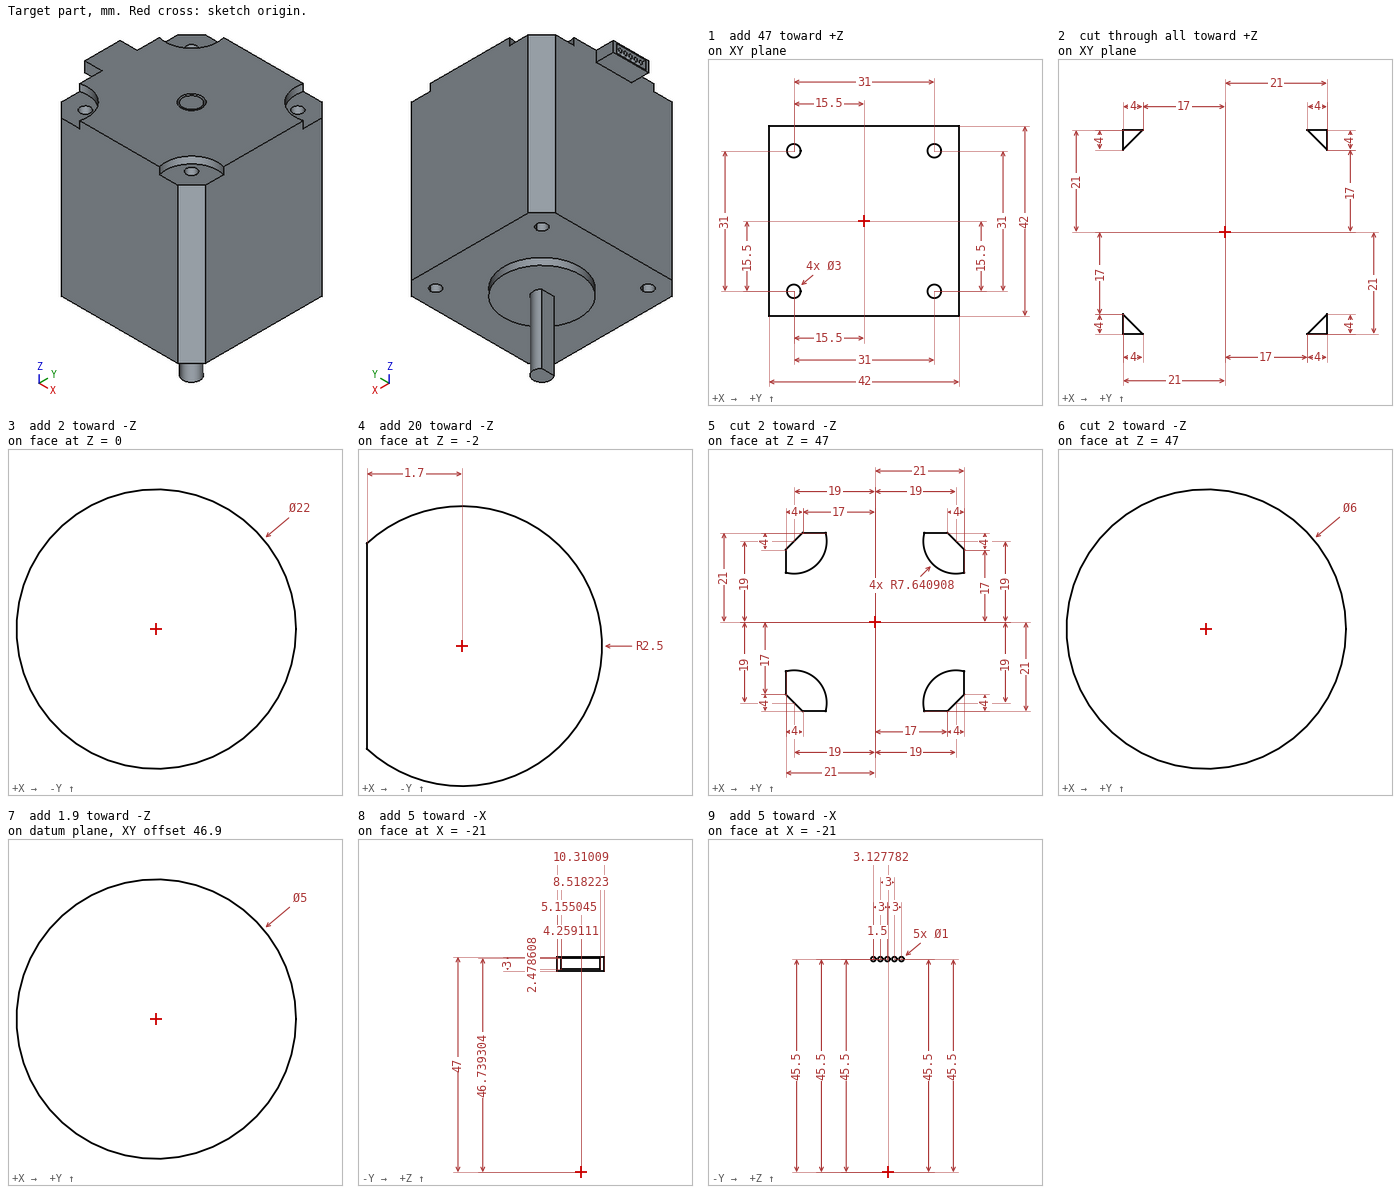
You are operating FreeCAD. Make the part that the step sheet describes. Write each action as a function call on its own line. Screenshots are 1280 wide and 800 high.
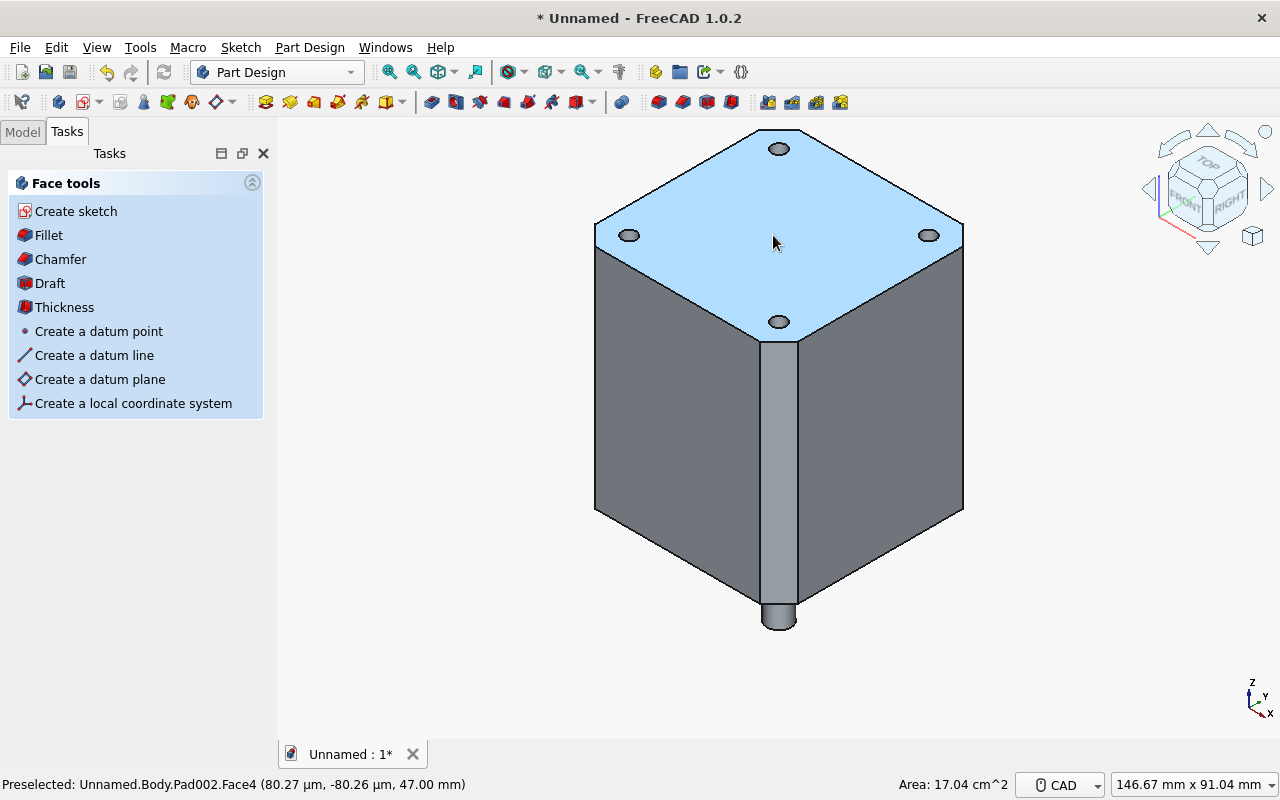
click(84, 102)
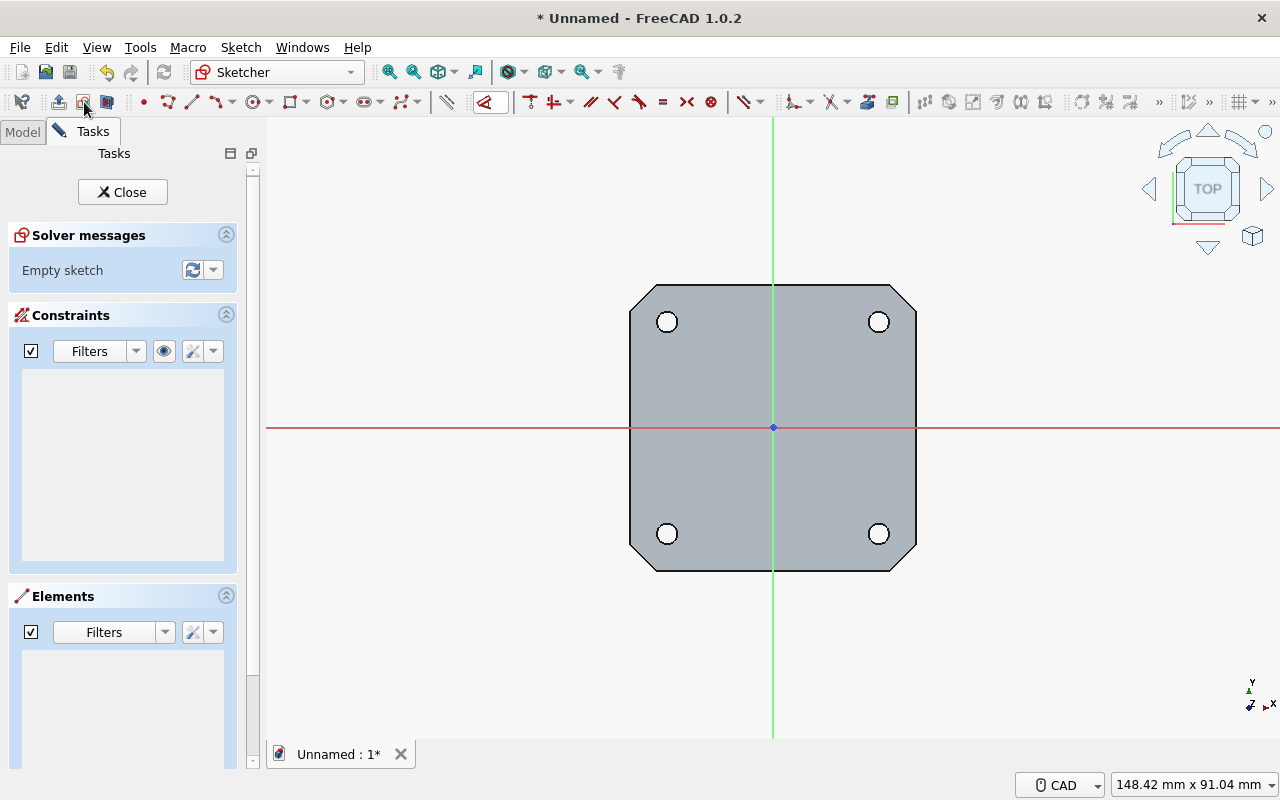
scroll(912, 428, up, 2)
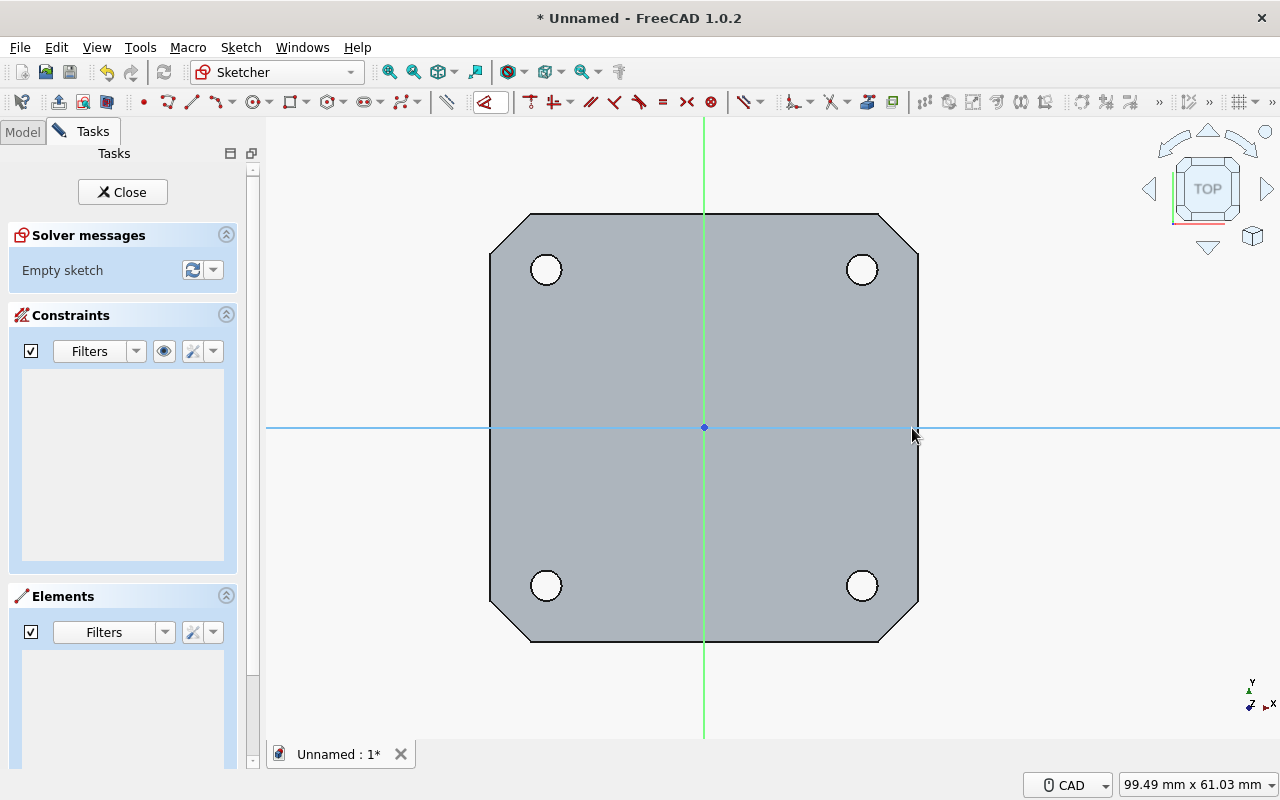
click(168, 102)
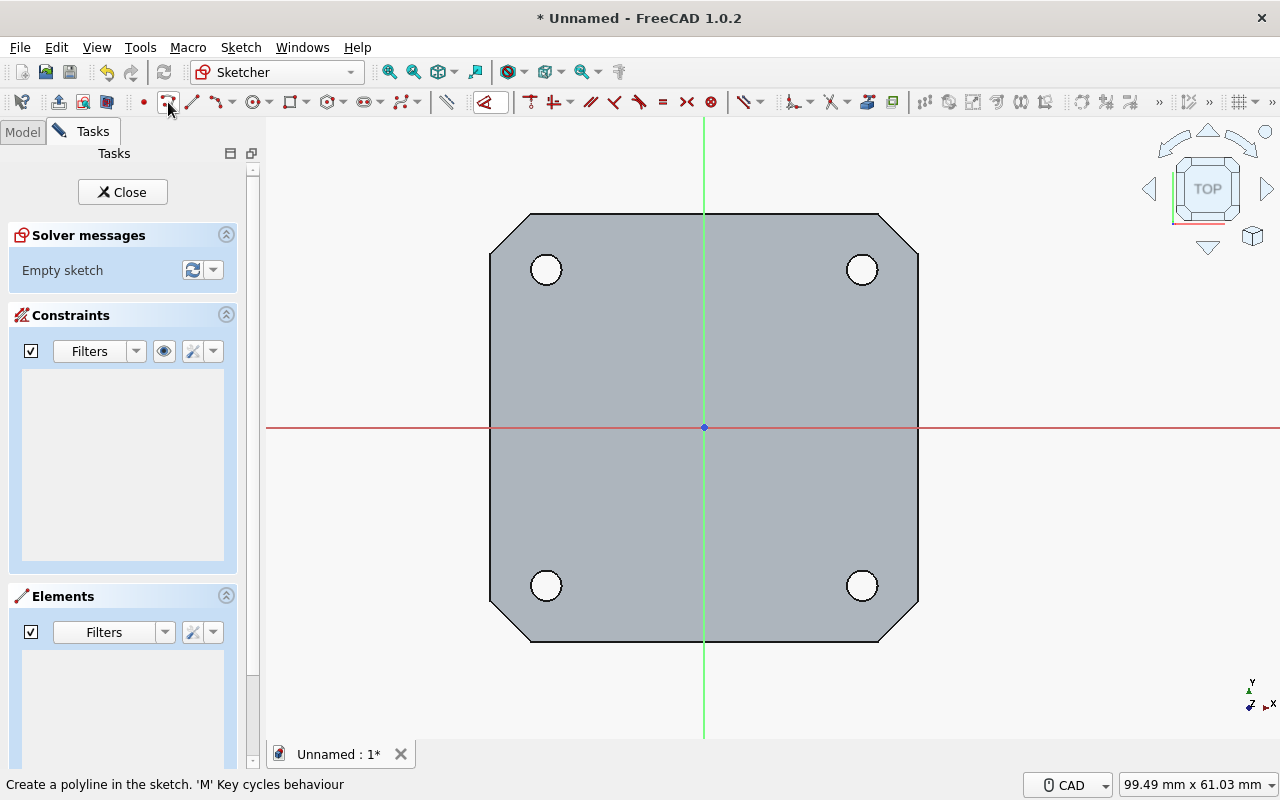
click(918, 309)
click(918, 254)
click(878, 214)
click(823, 214)
right_click(823, 214)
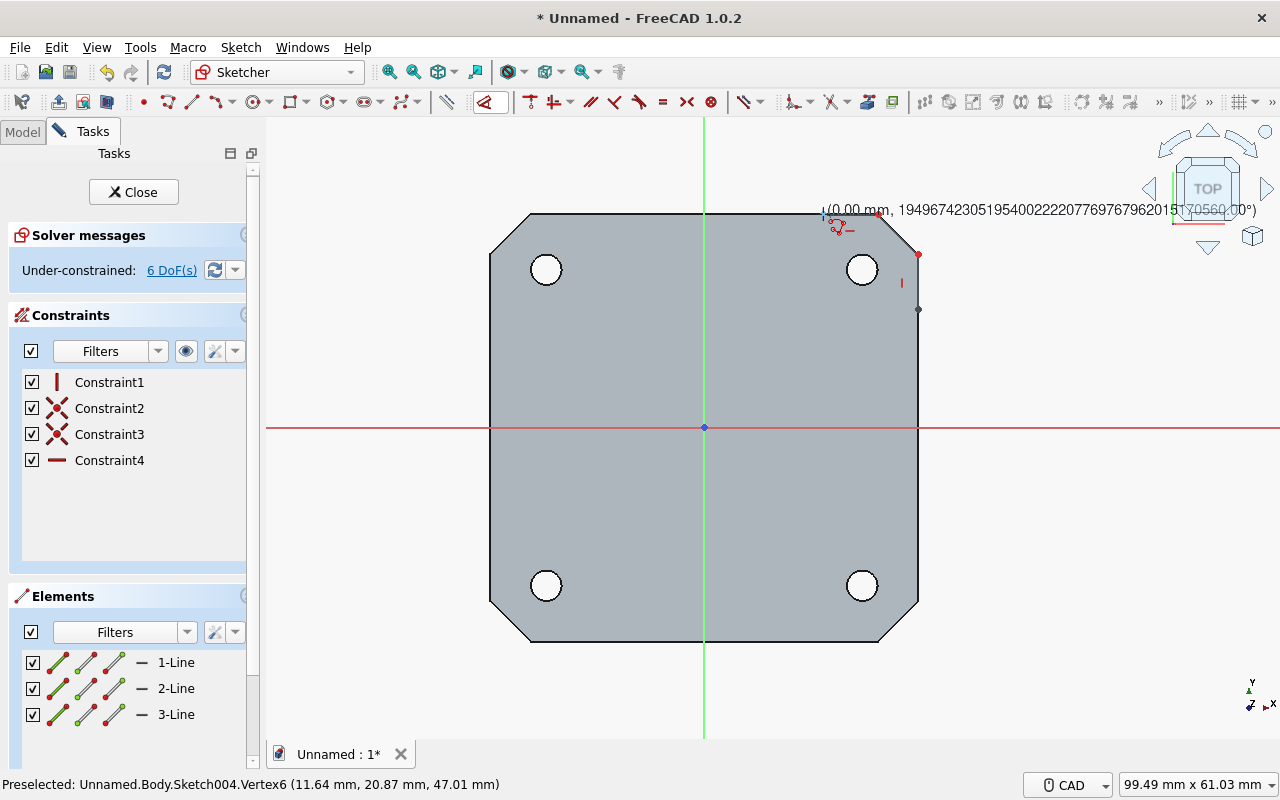
click(216, 102)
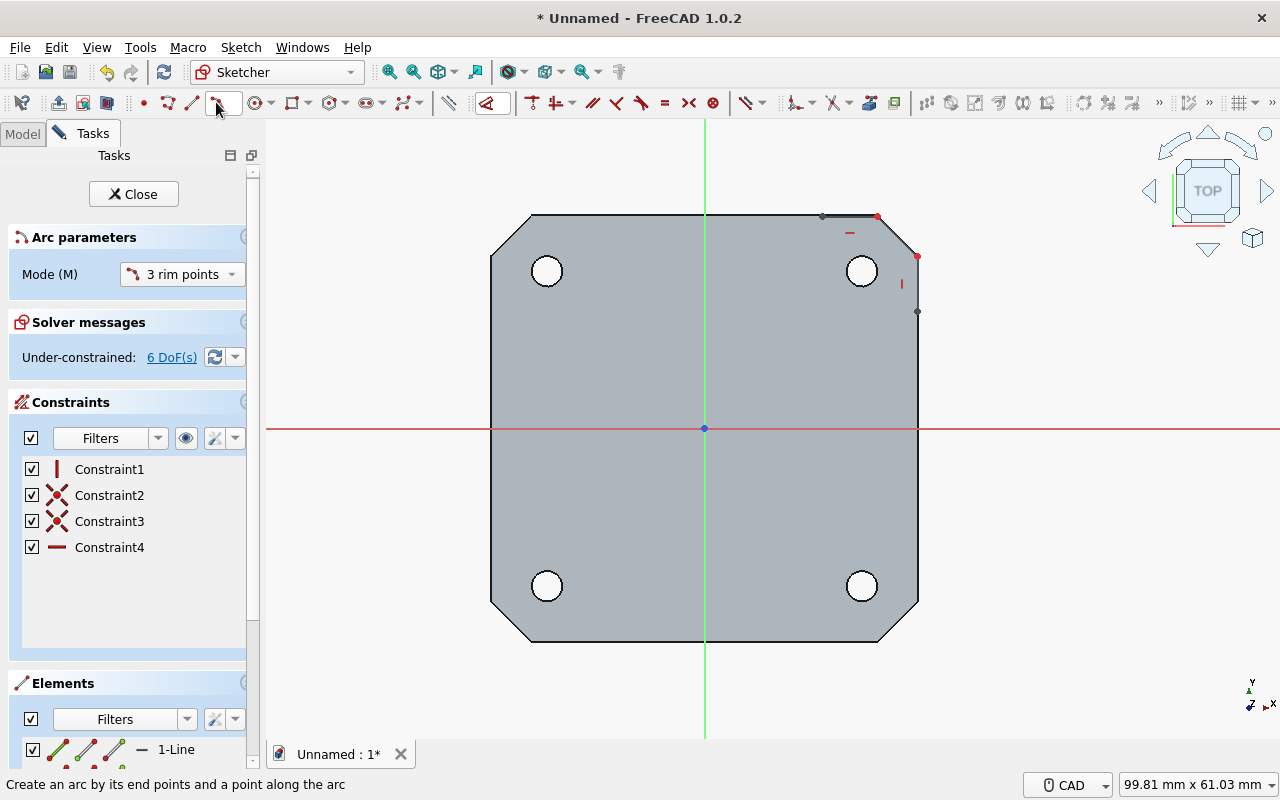
click(823, 217)
click(918, 311)
click(843, 291)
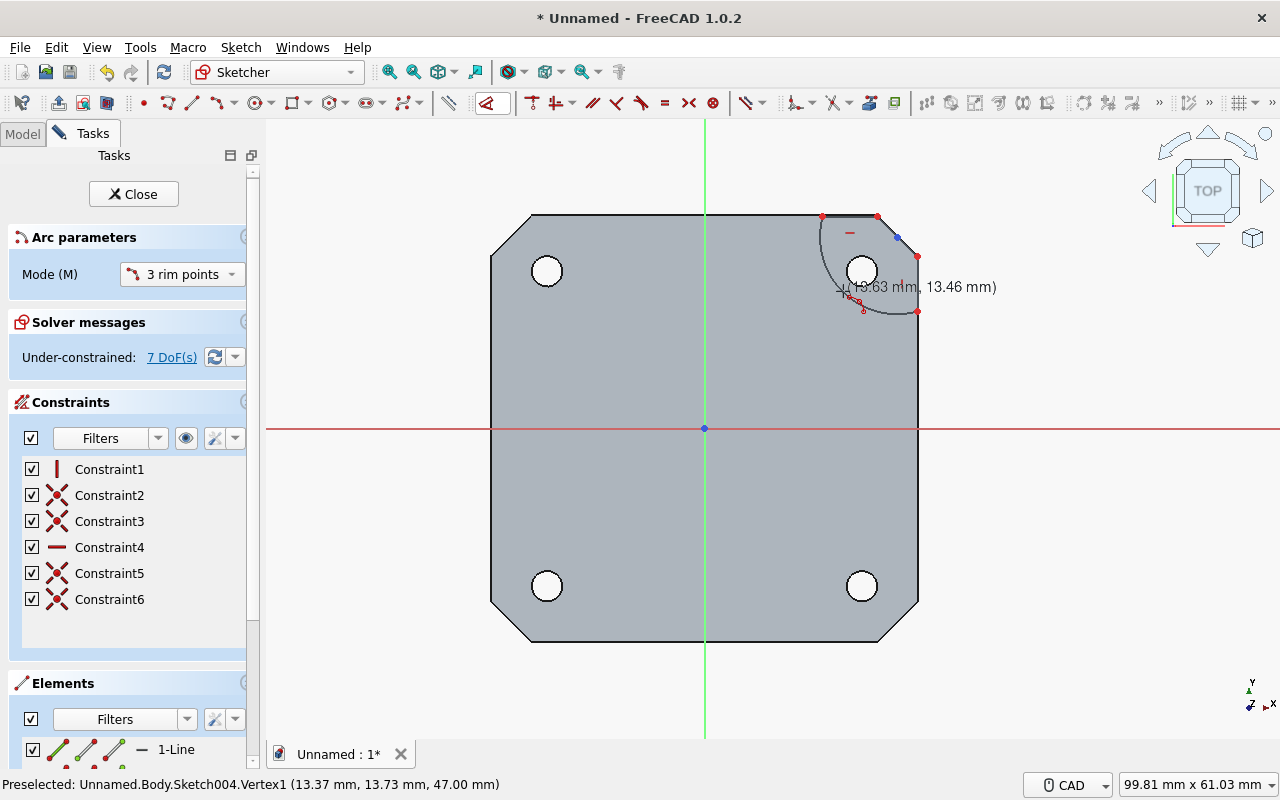
key(g)
key(m)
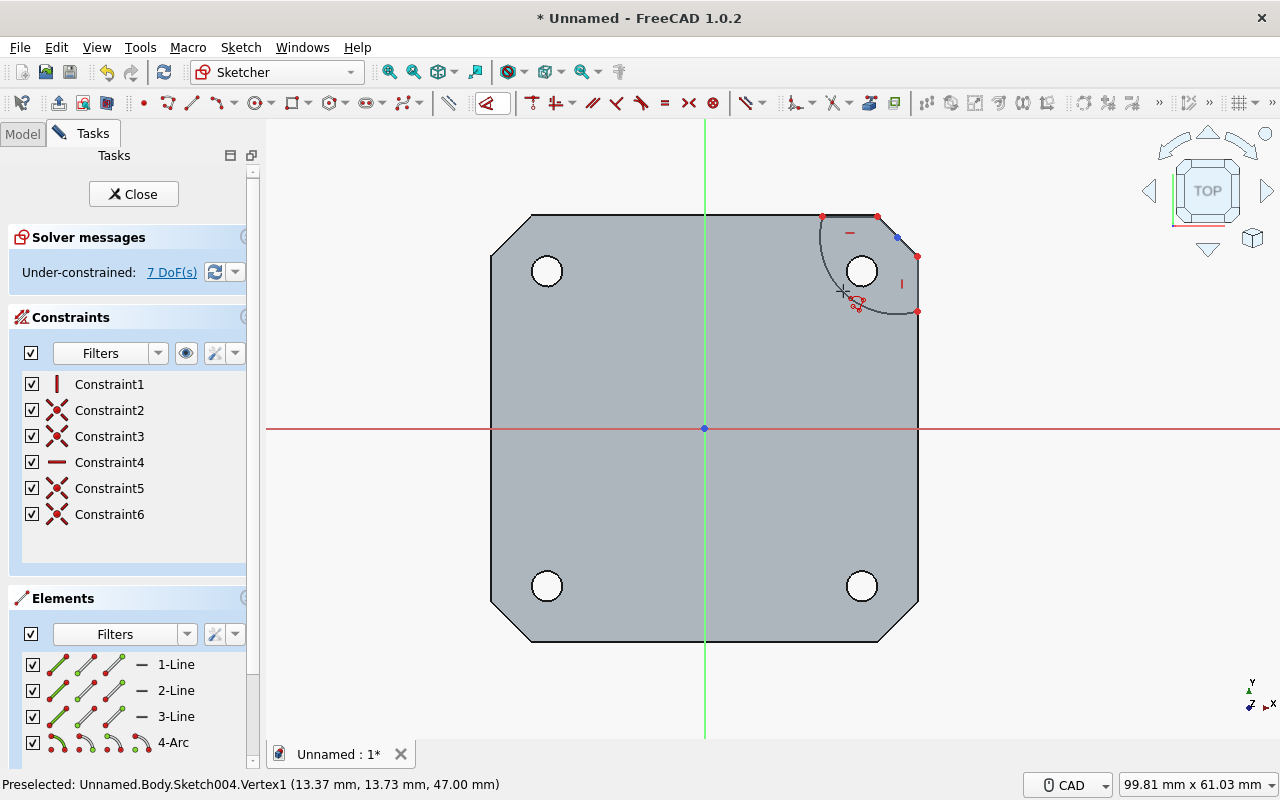
click(491, 547)
click(491, 601)
click(532, 642)
click(586, 642)
right_click(586, 642)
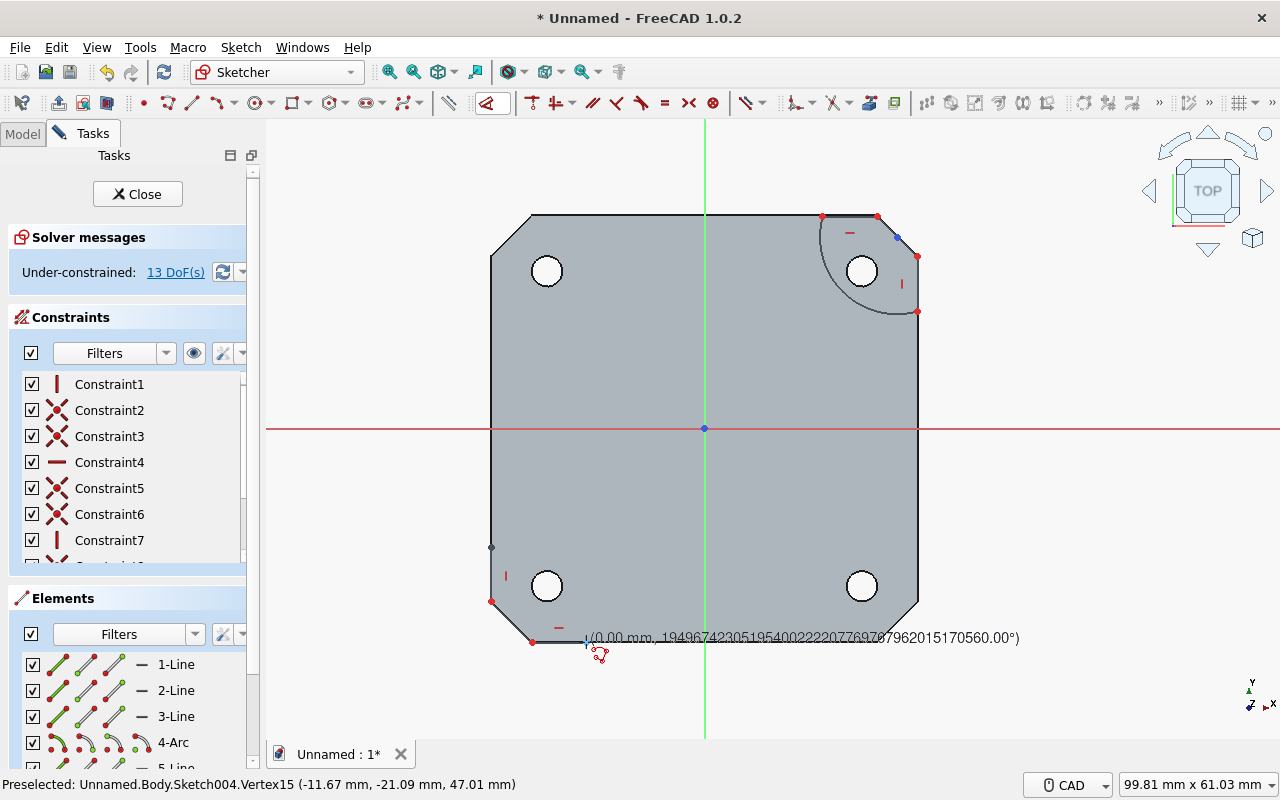
key(g)
key(3)
key(a)